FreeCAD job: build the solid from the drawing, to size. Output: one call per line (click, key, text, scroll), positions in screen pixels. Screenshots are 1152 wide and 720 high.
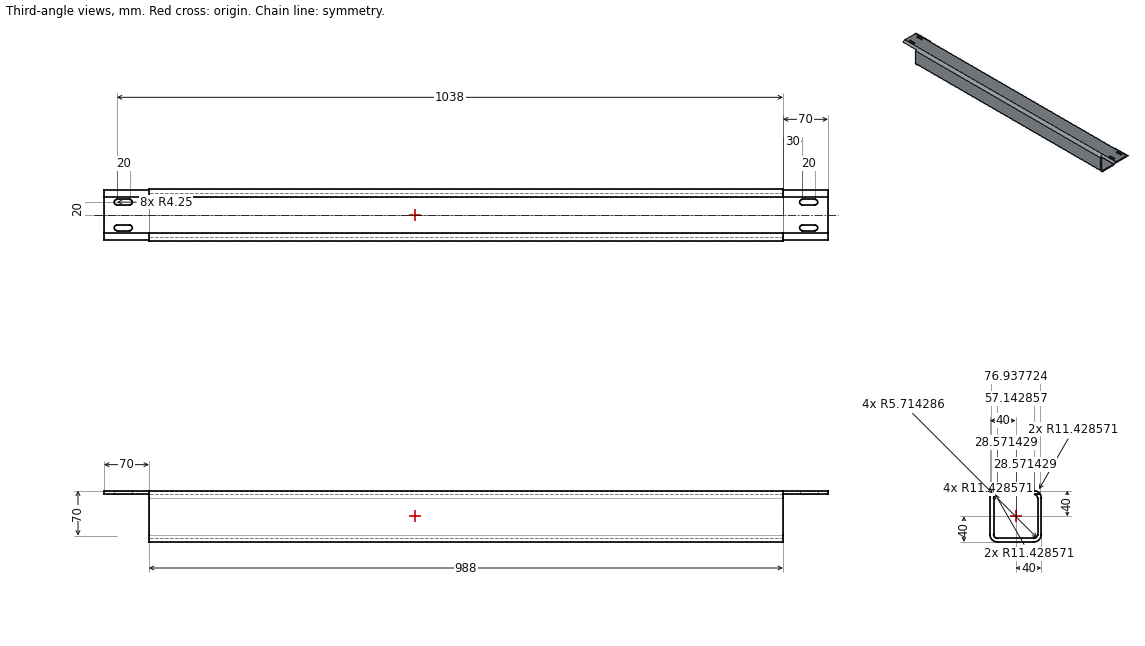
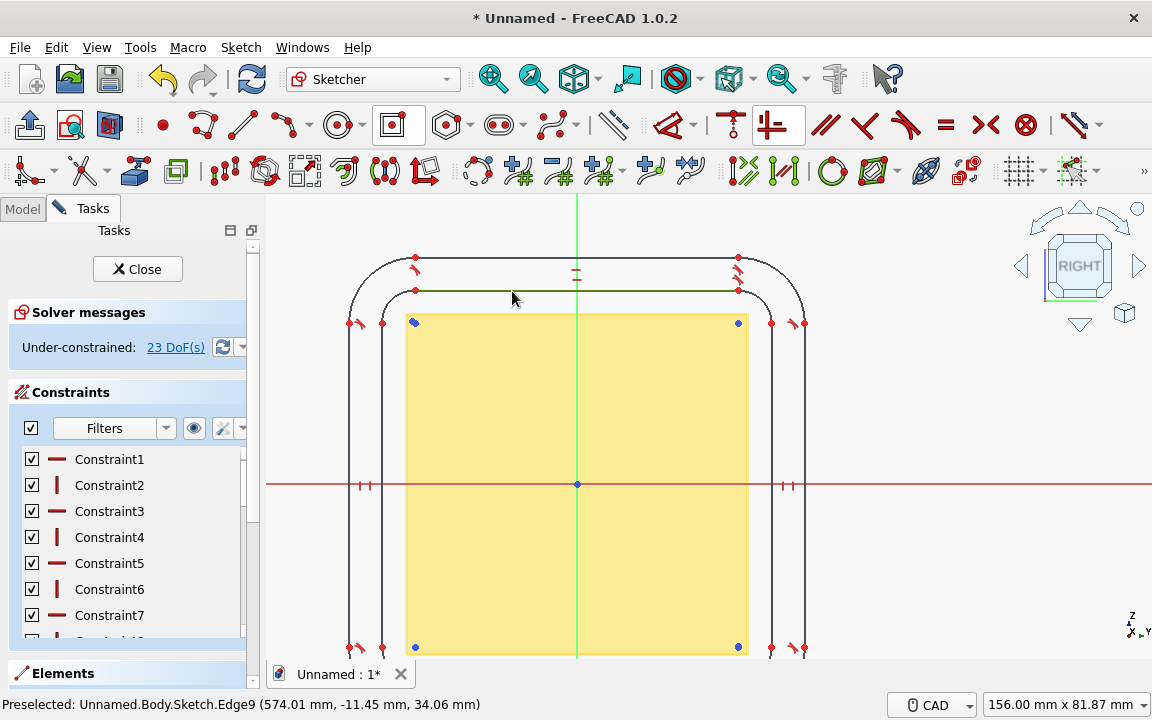
click(400, 294)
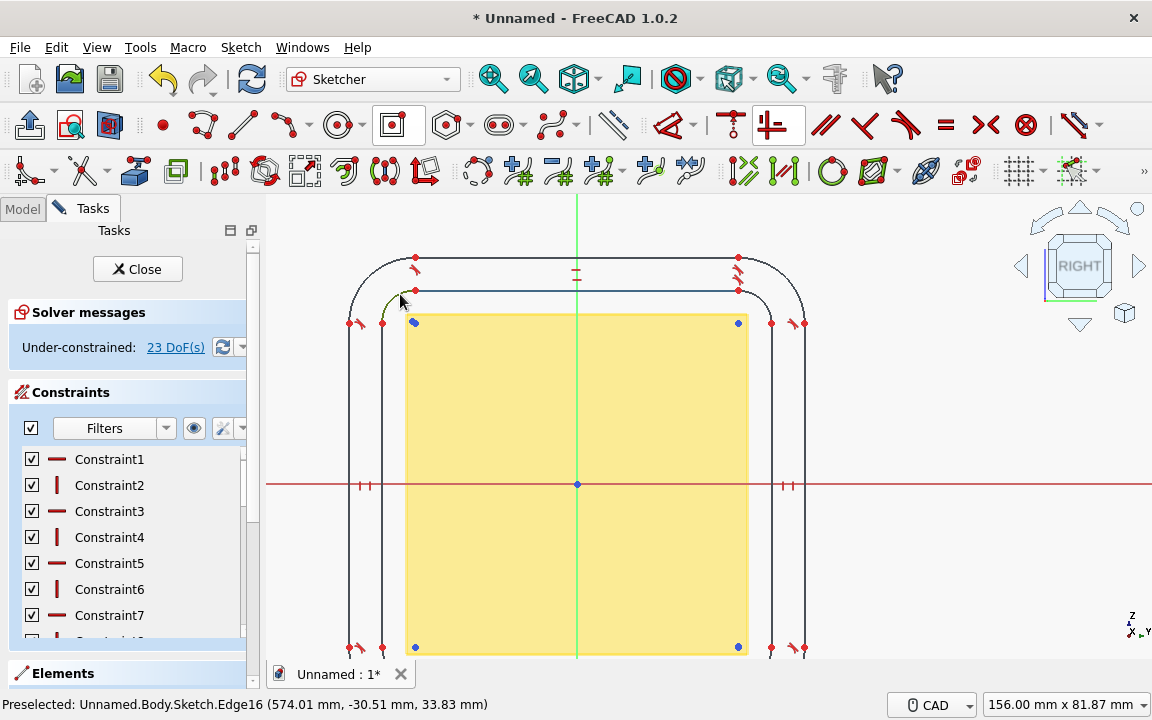
key(t)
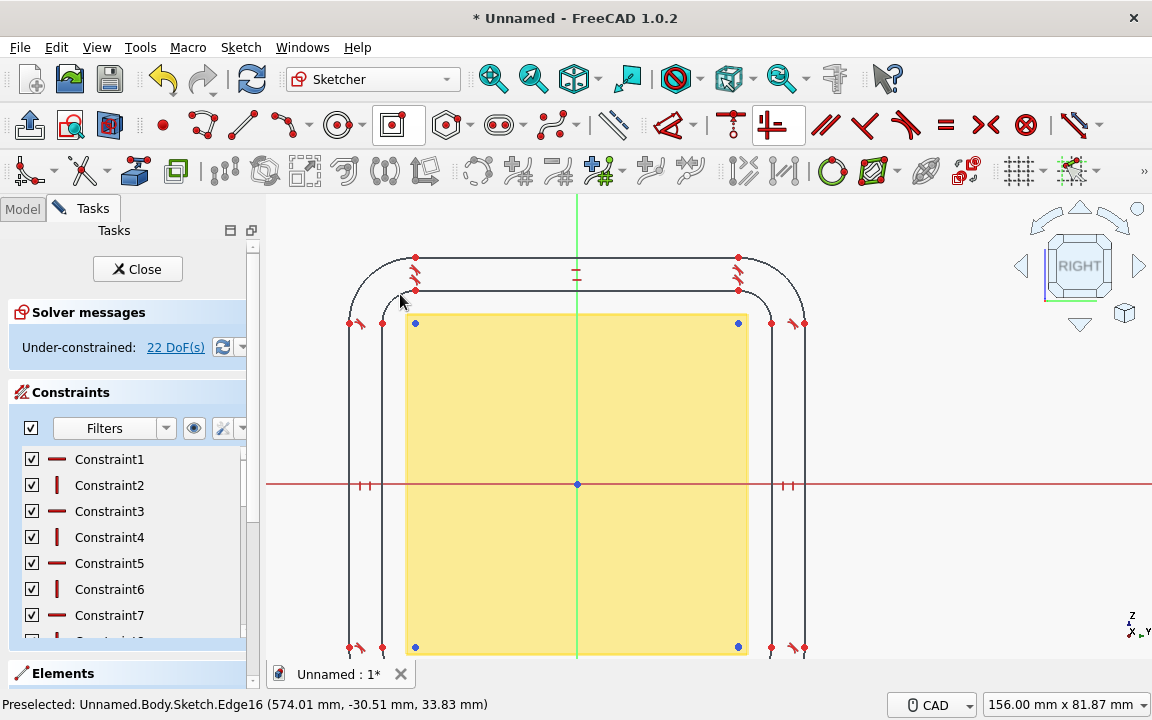
click(772, 421)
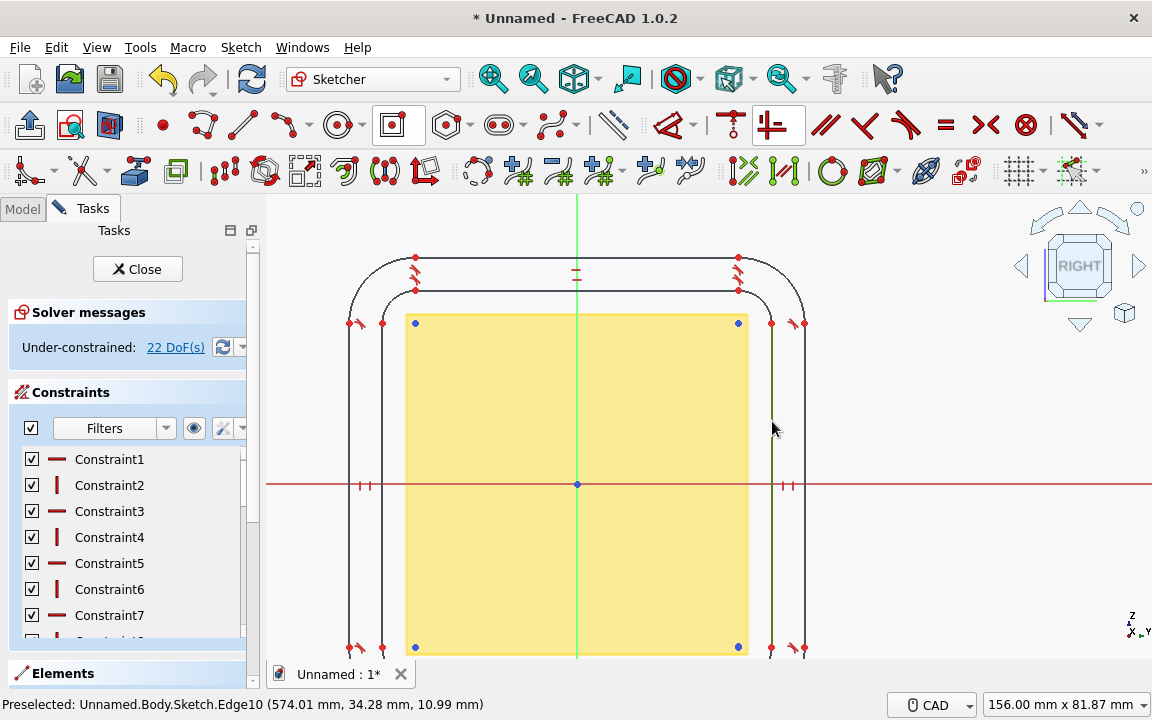
click(768, 309)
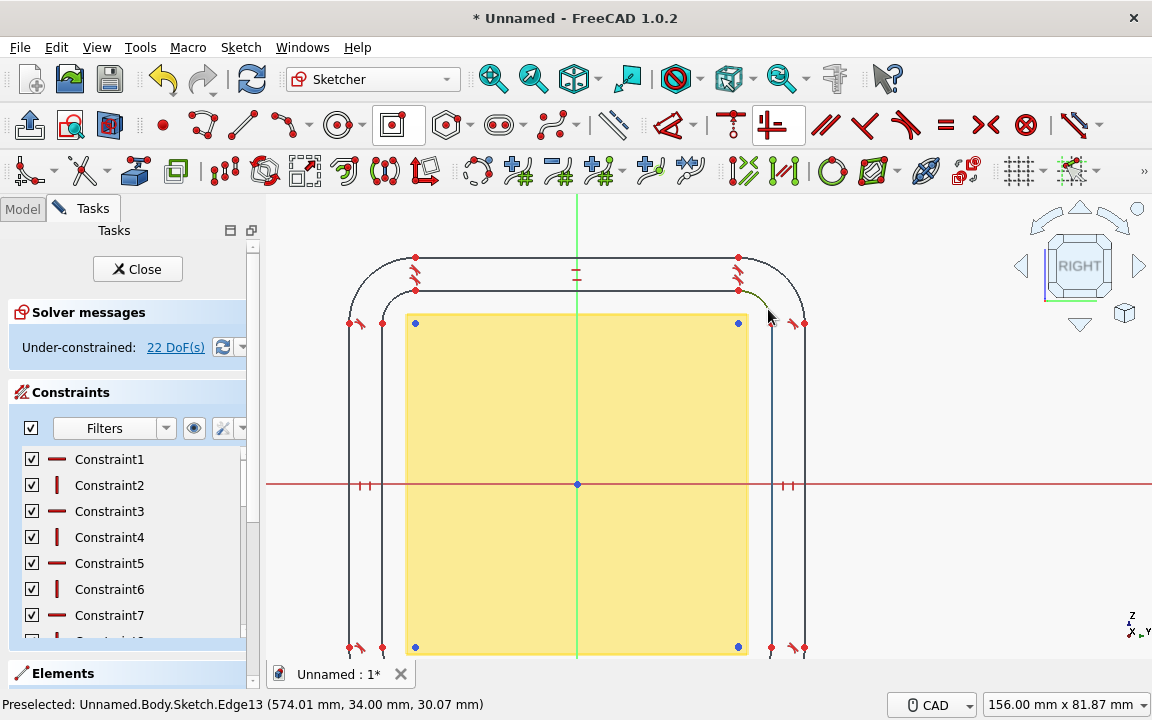
key(t)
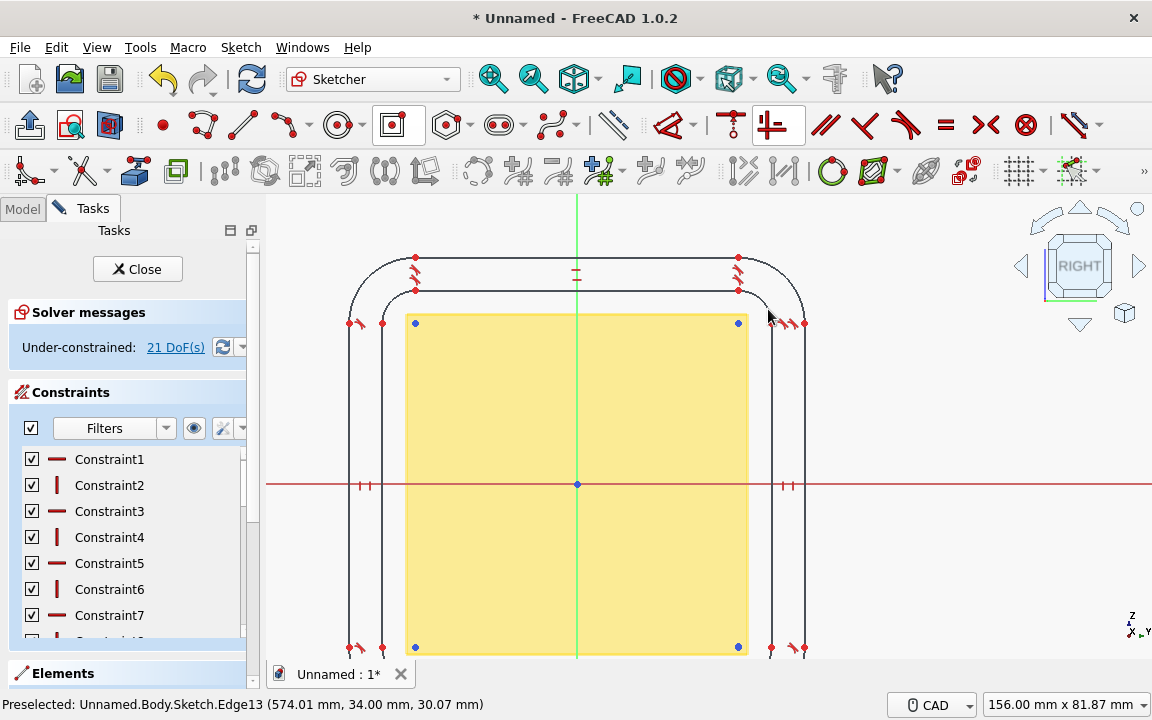
click(772, 421)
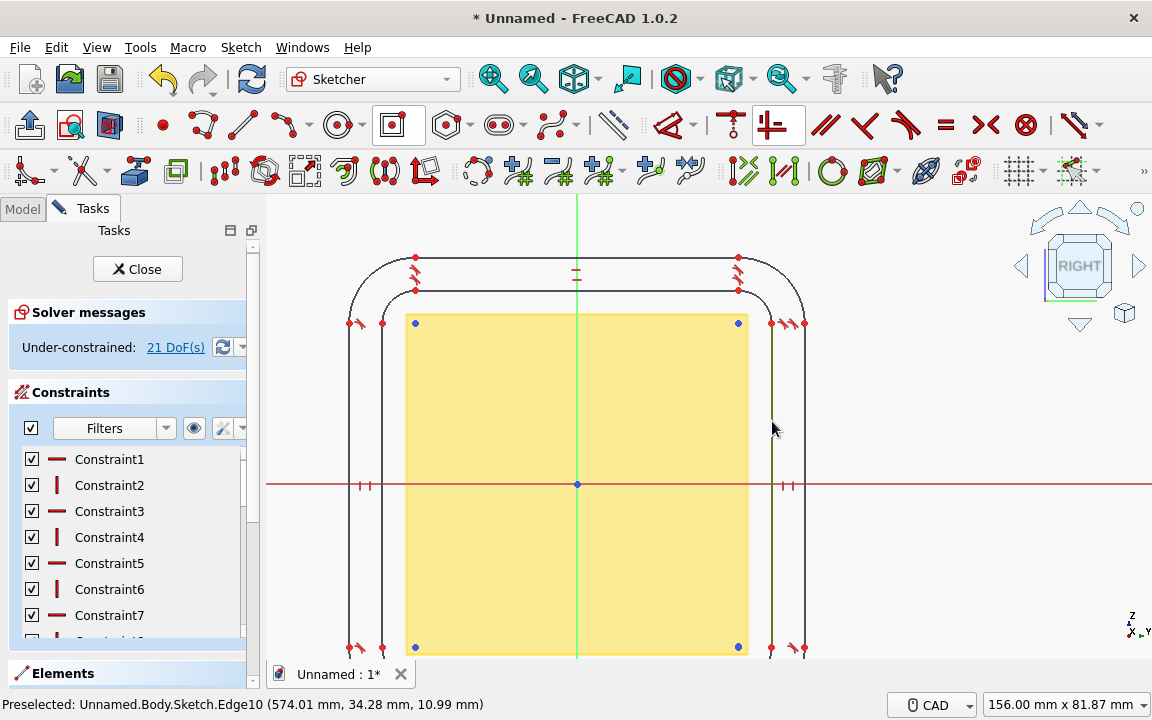
scroll(770, 309, down, 2)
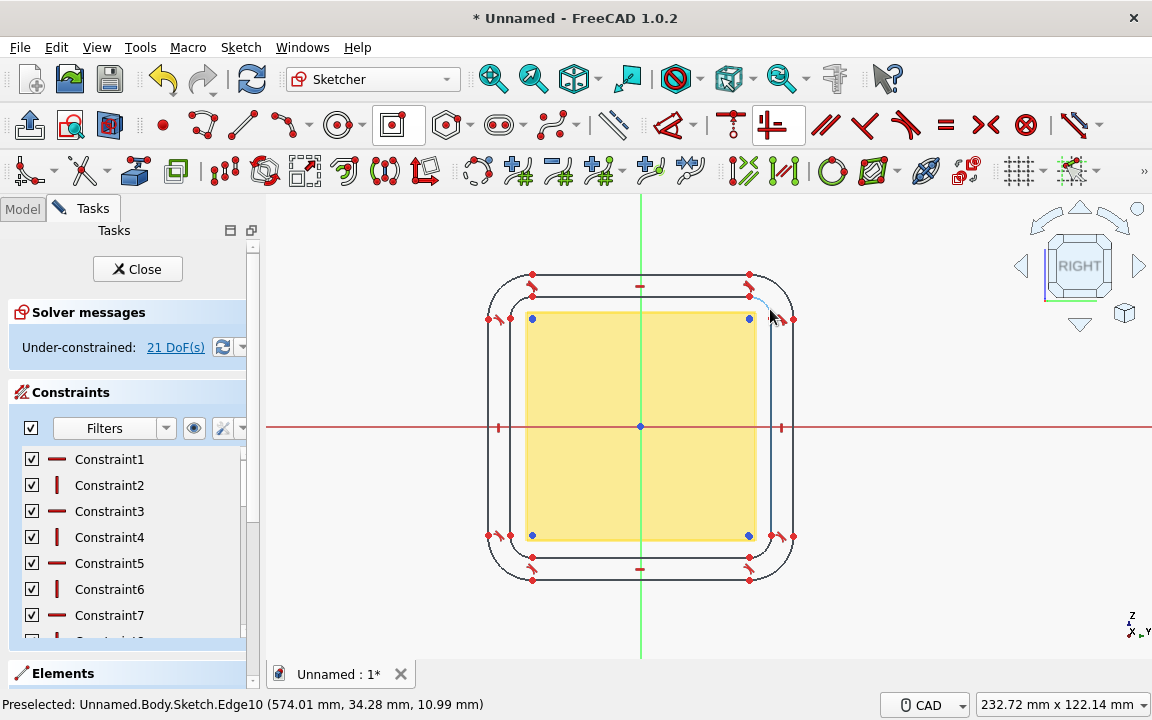
scroll(759, 555, up, 2)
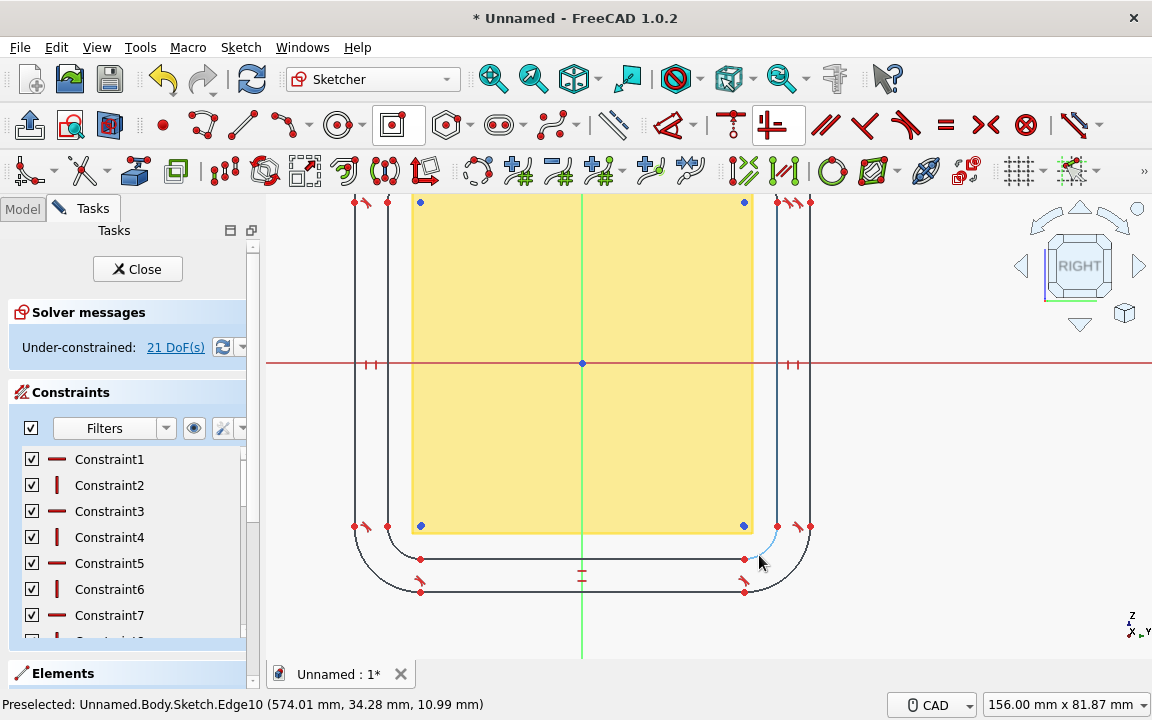
click(759, 555)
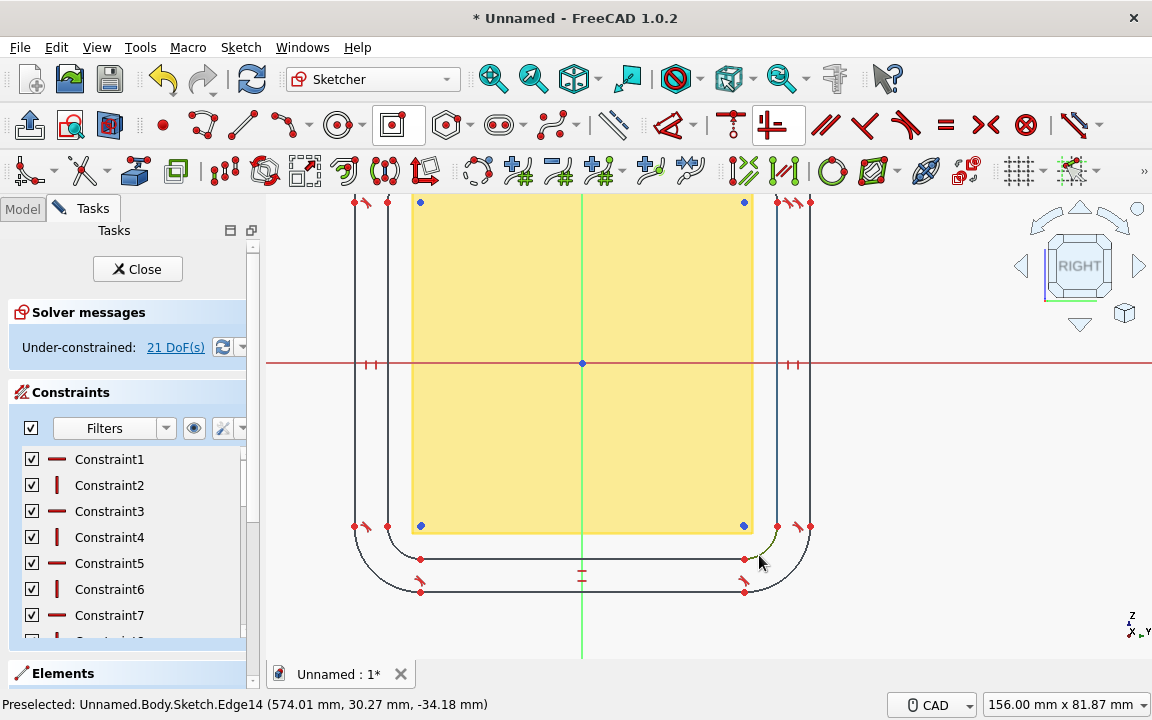
key(t)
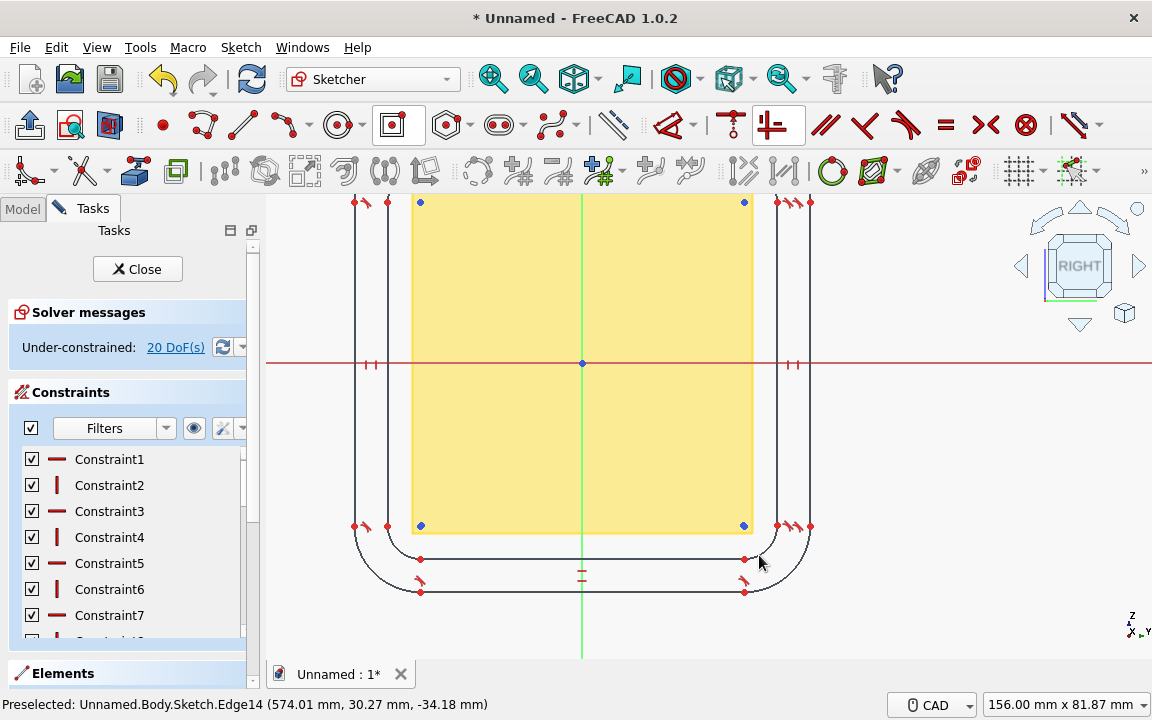
click(647, 559)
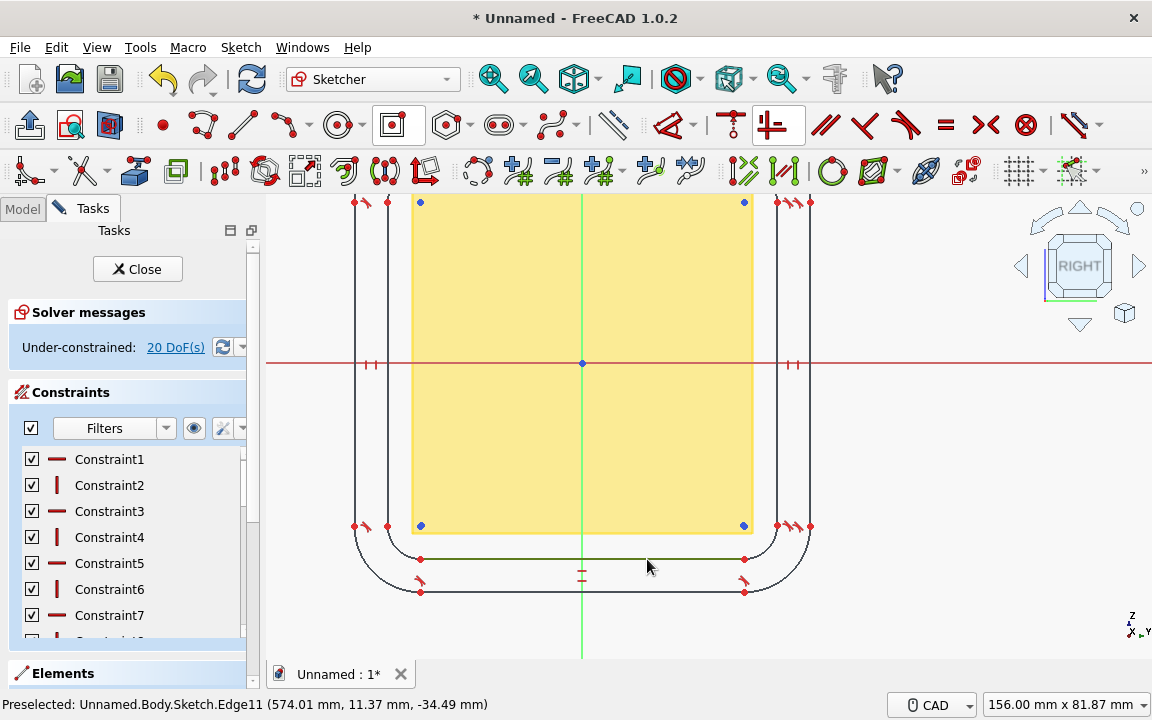
click(759, 555)